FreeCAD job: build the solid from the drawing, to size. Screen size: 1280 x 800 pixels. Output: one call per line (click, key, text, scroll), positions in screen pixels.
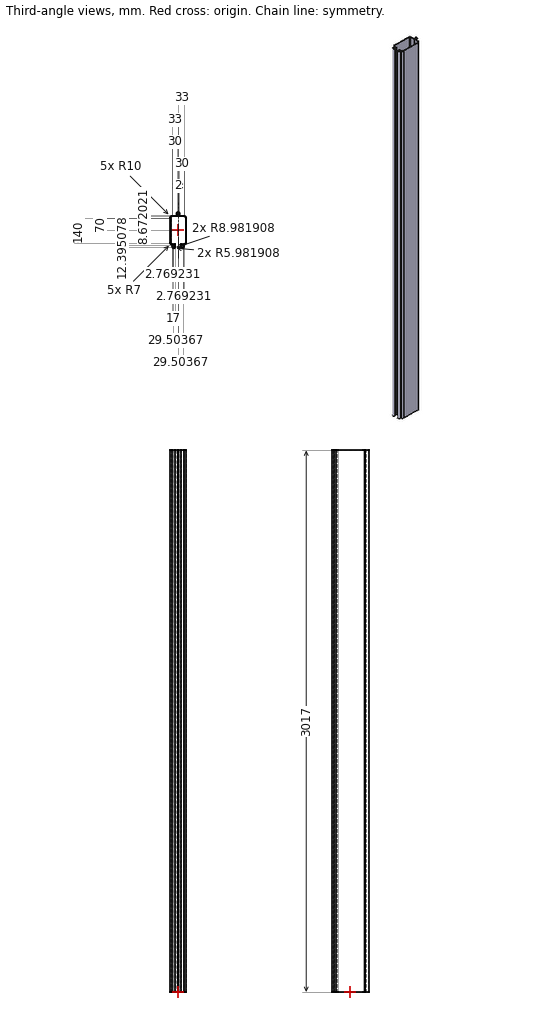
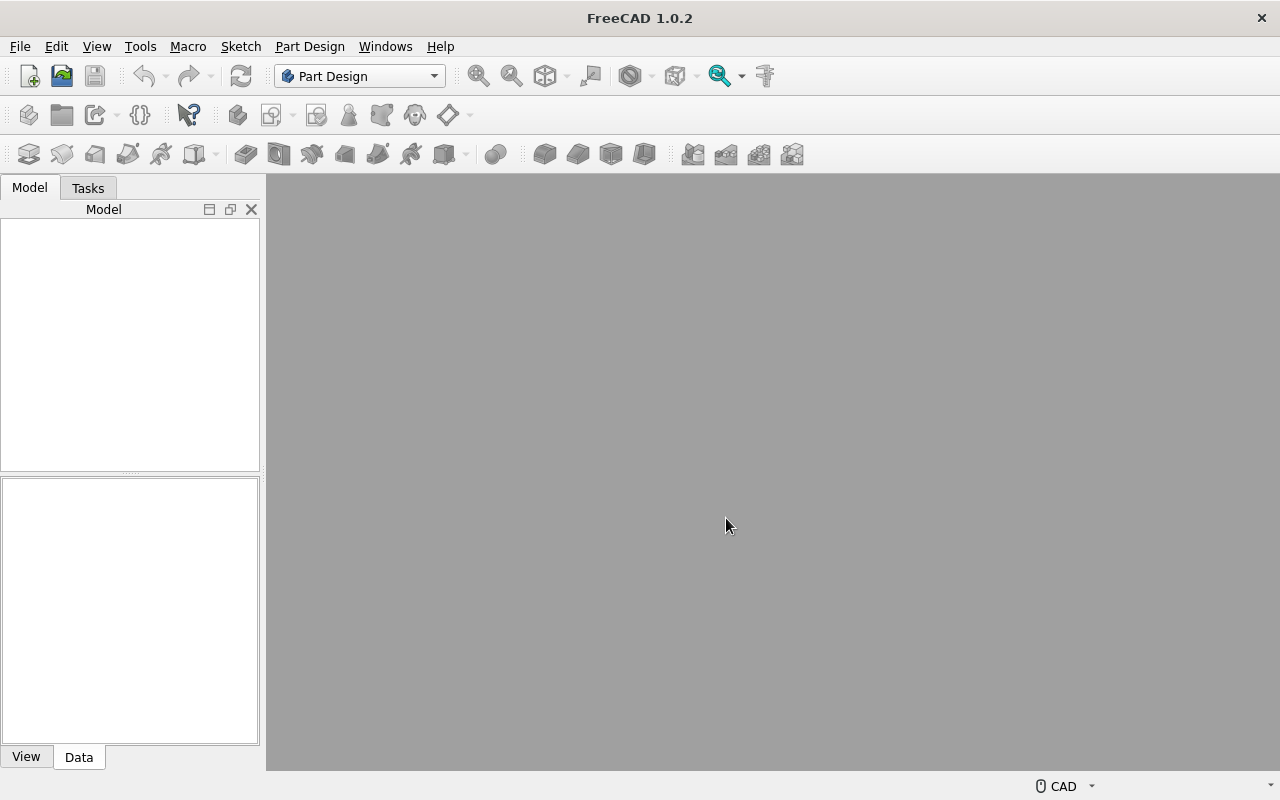
click(29, 76)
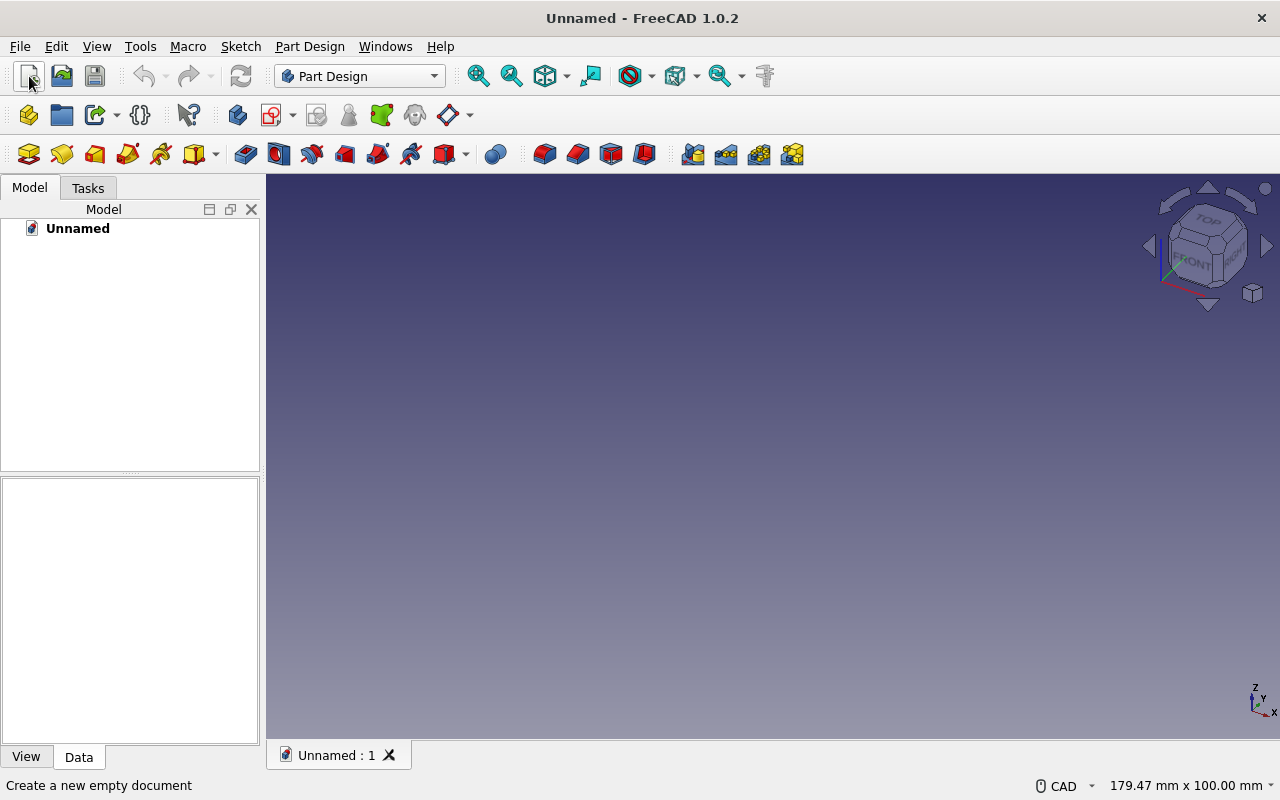
click(270, 116)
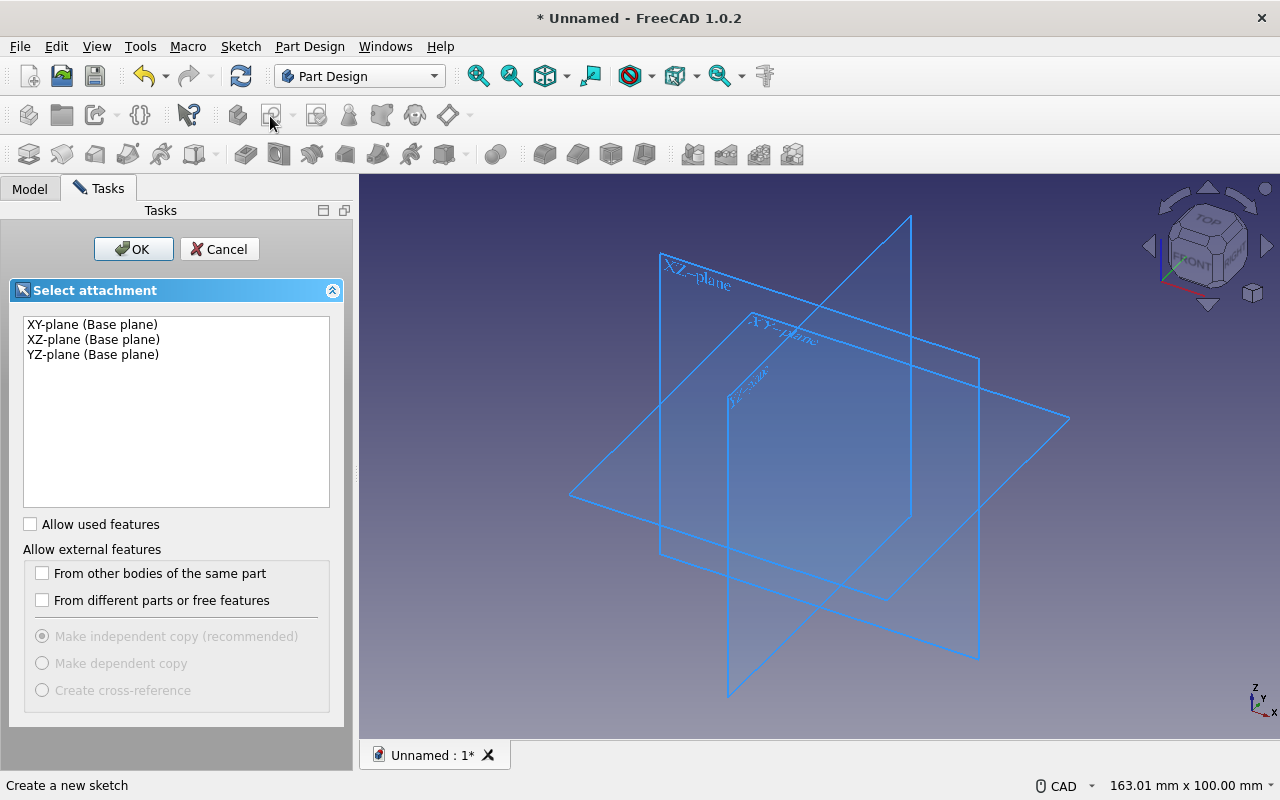
click(84, 324)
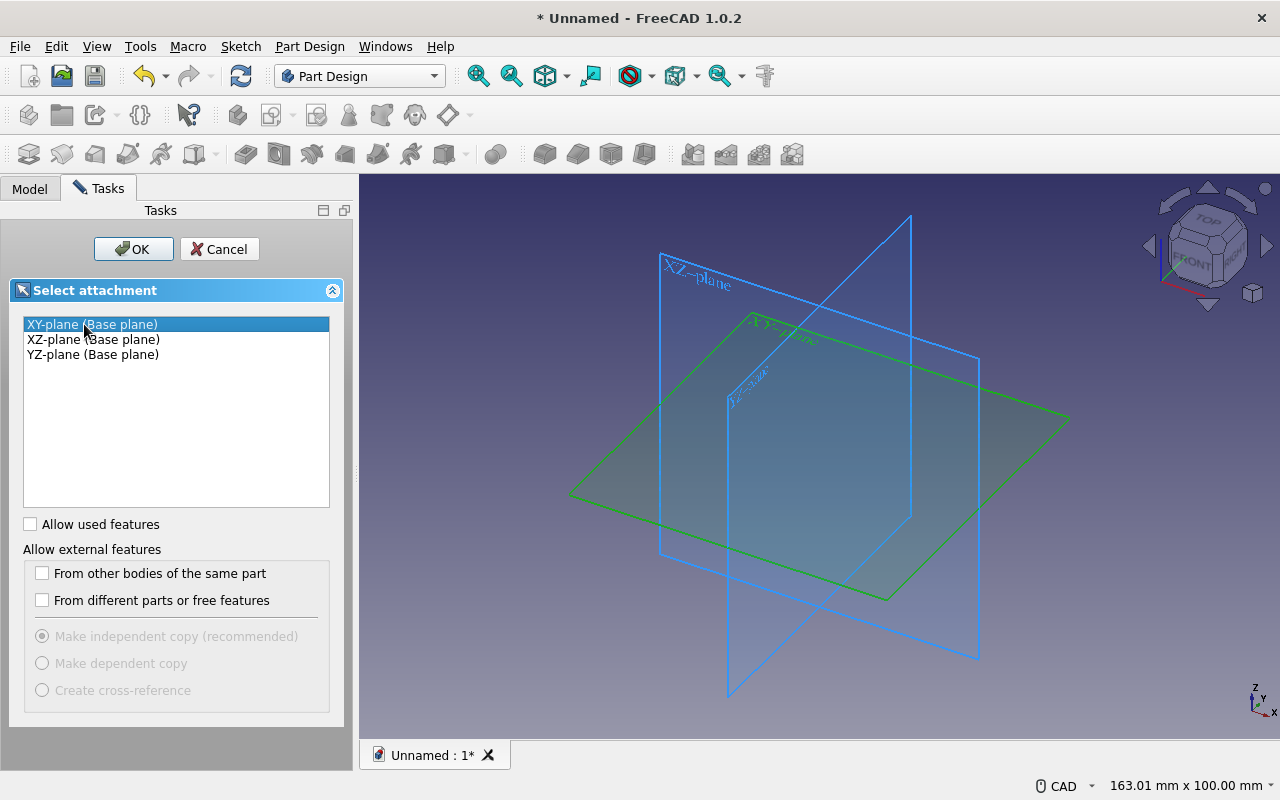
click(134, 249)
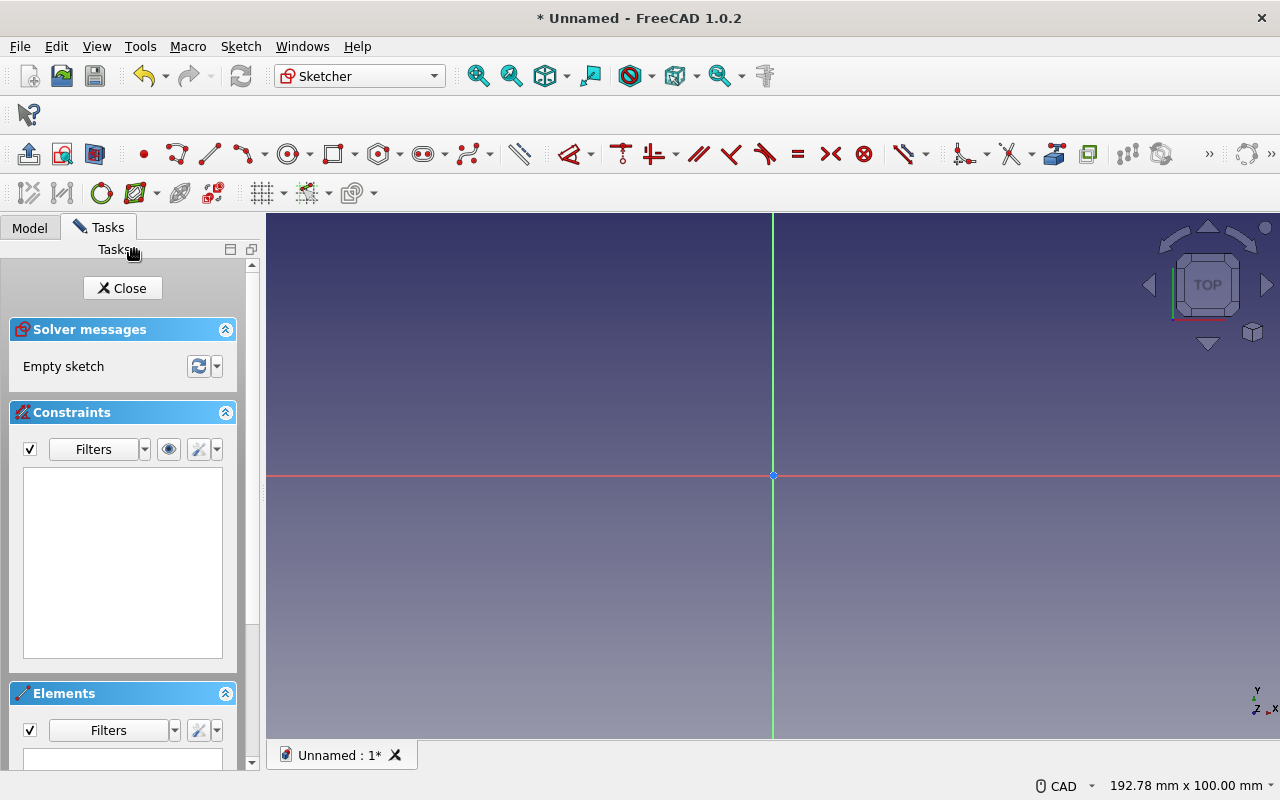
scroll(675, 477, down, 6)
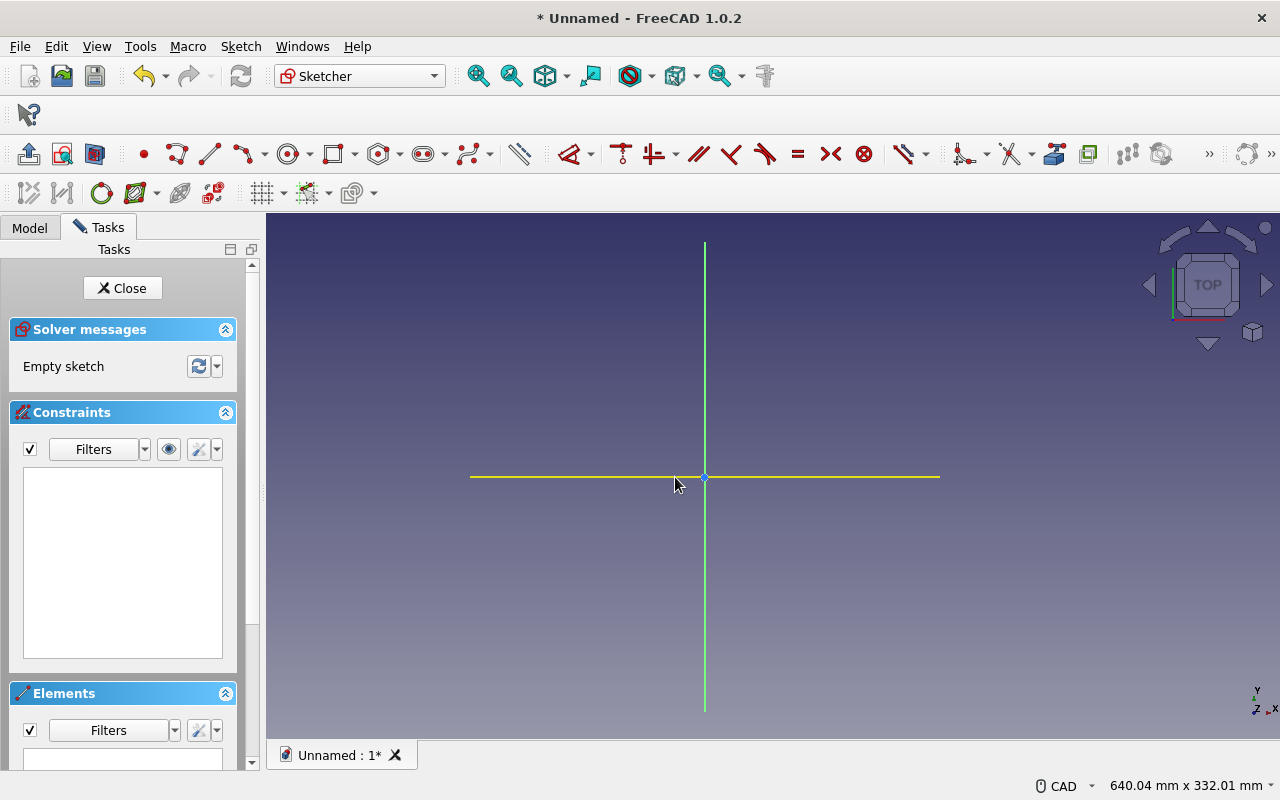
click(210, 154)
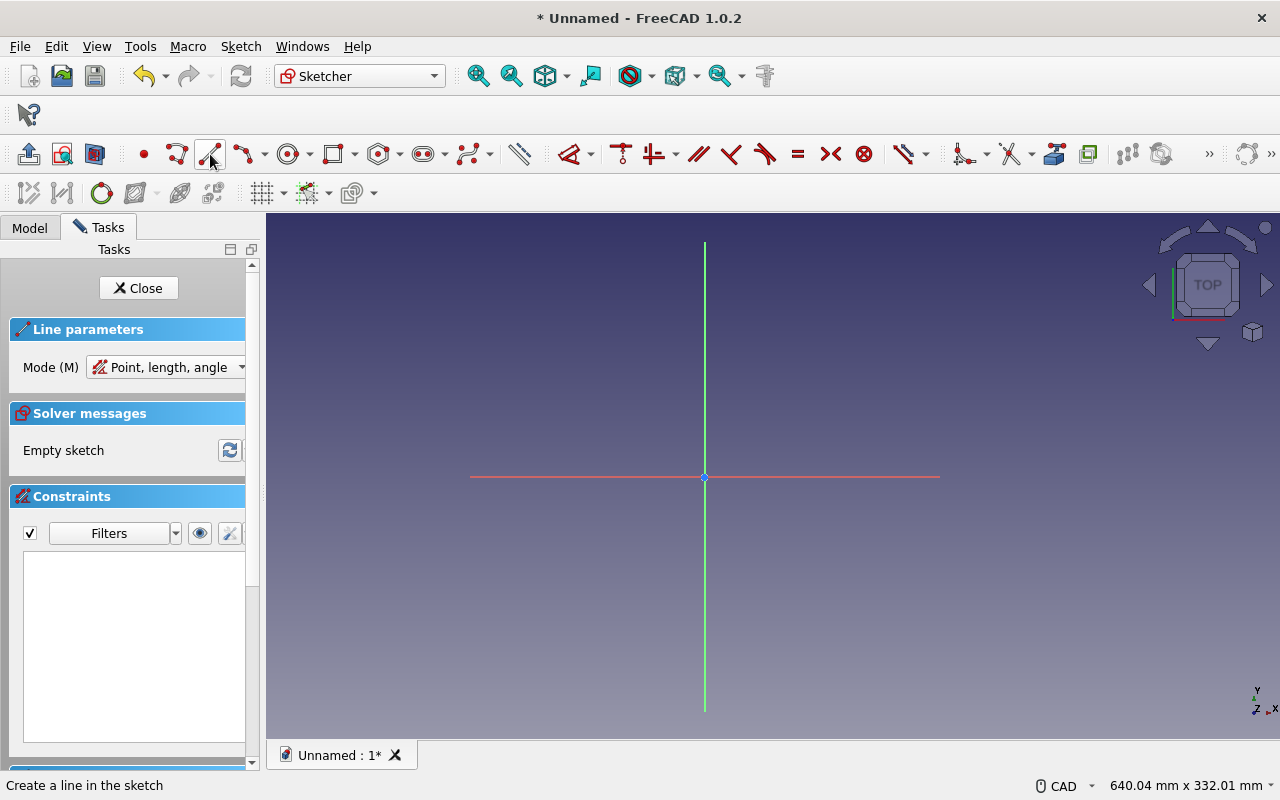
click(634, 366)
click(634, 588)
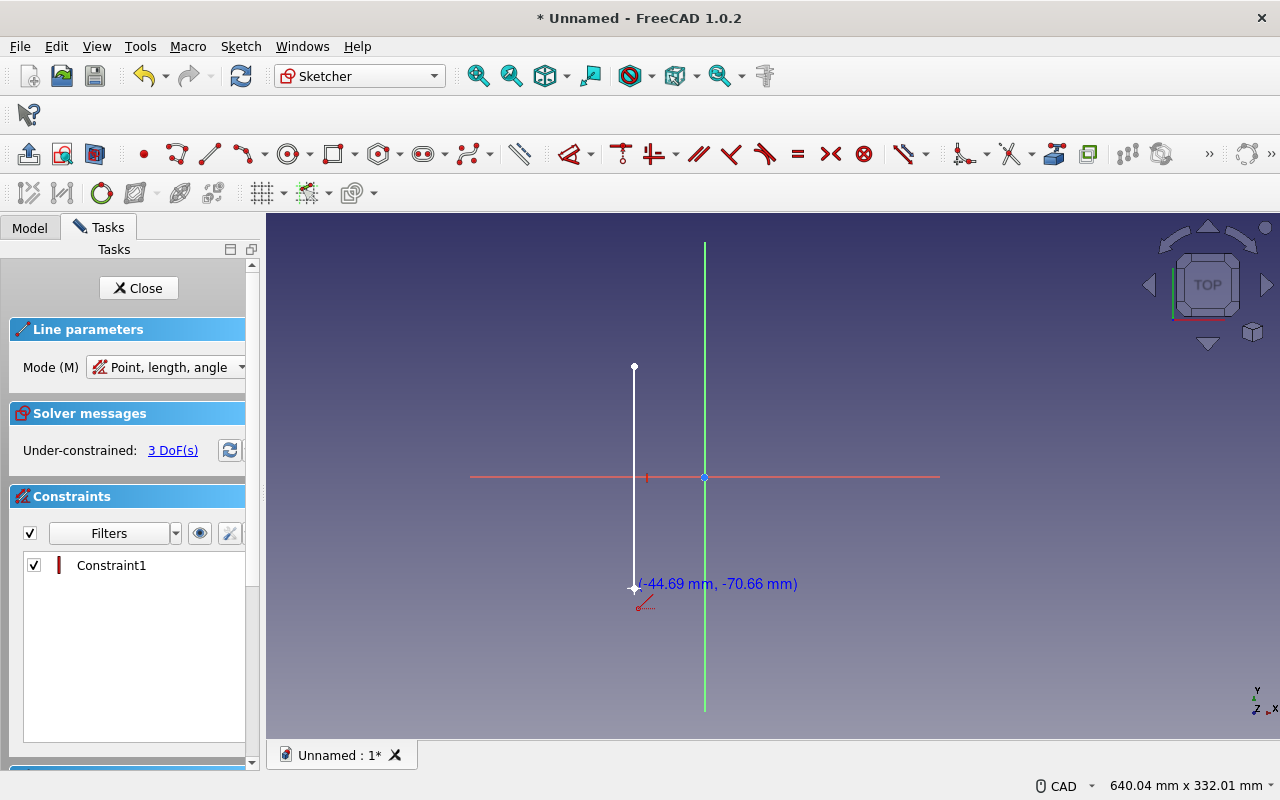
click(177, 154)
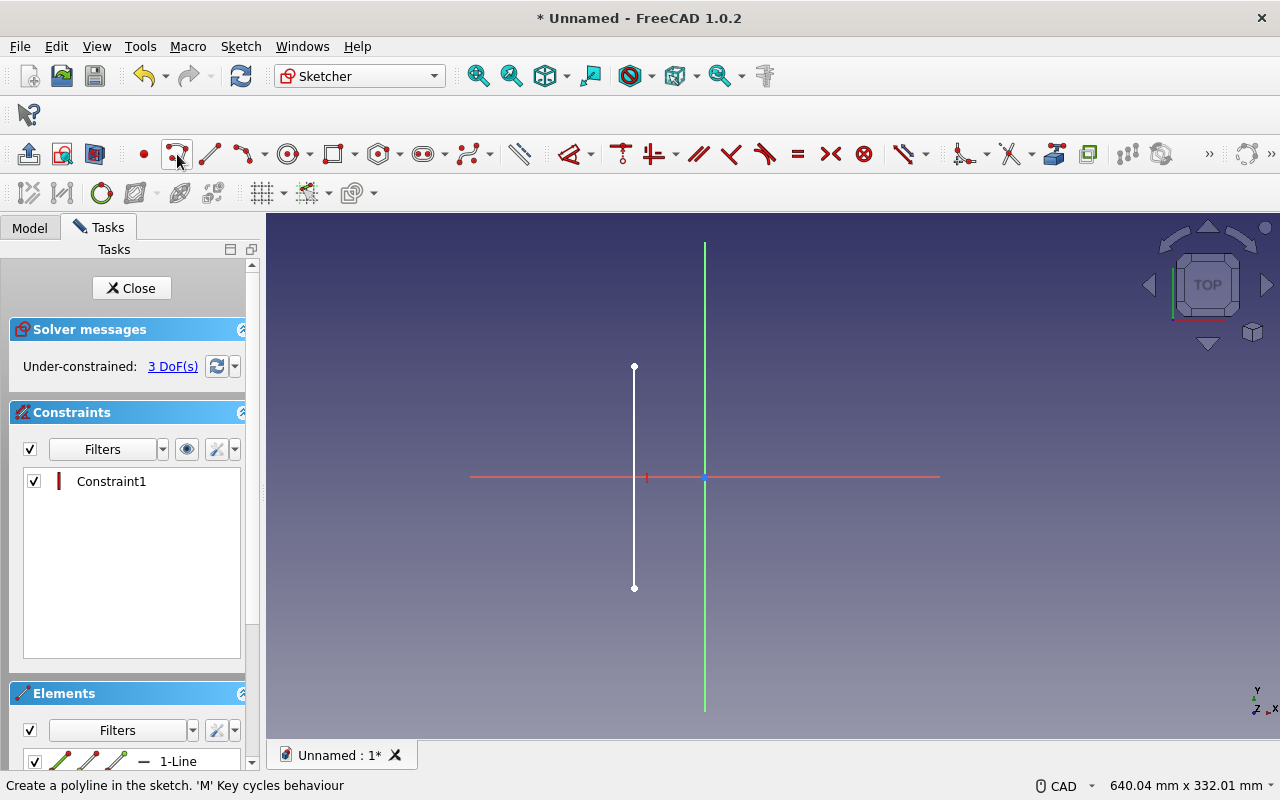
click(649, 604)
click(676, 604)
click(676, 623)
right_click(676, 623)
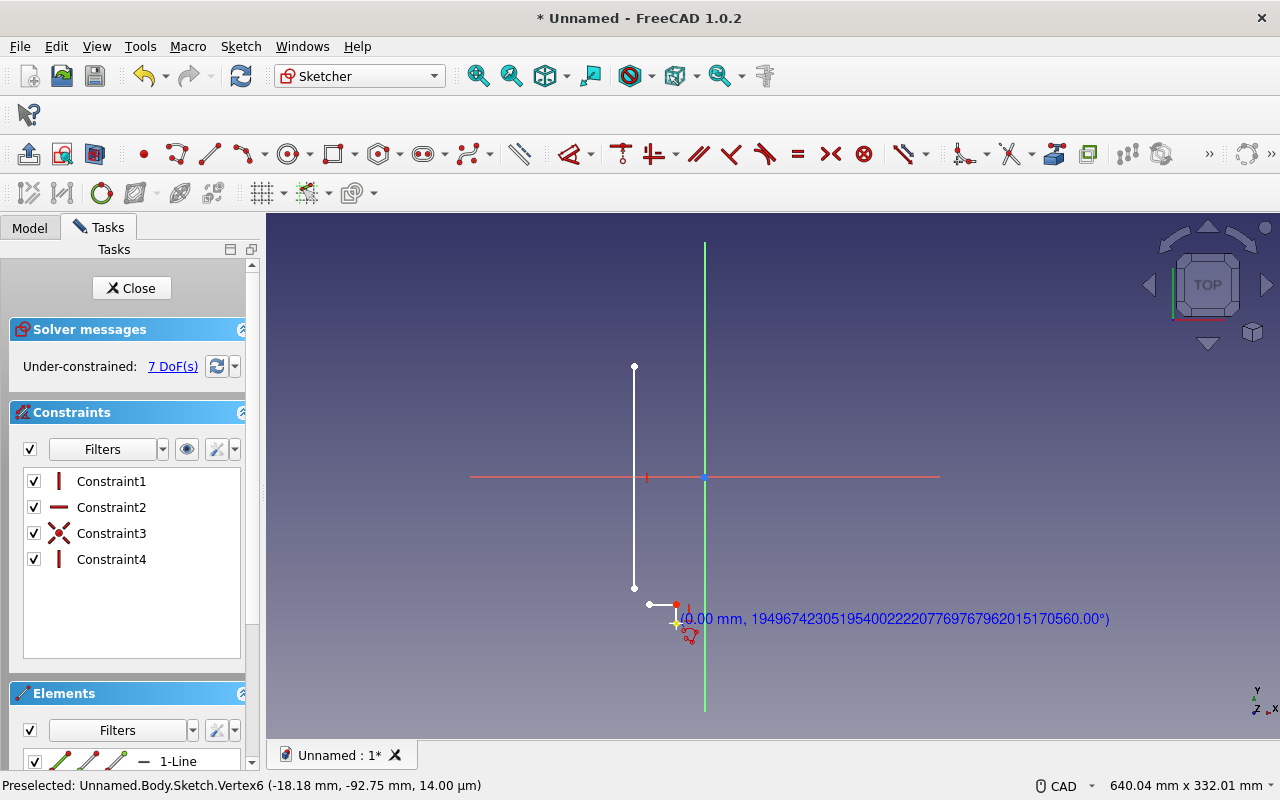
click(210, 154)